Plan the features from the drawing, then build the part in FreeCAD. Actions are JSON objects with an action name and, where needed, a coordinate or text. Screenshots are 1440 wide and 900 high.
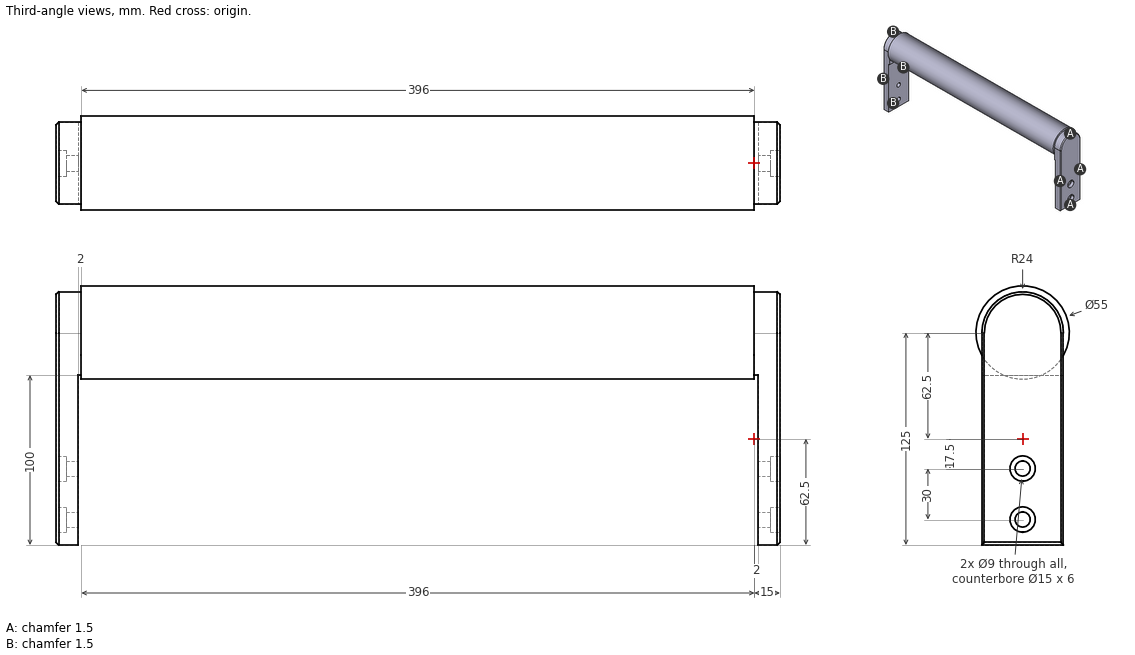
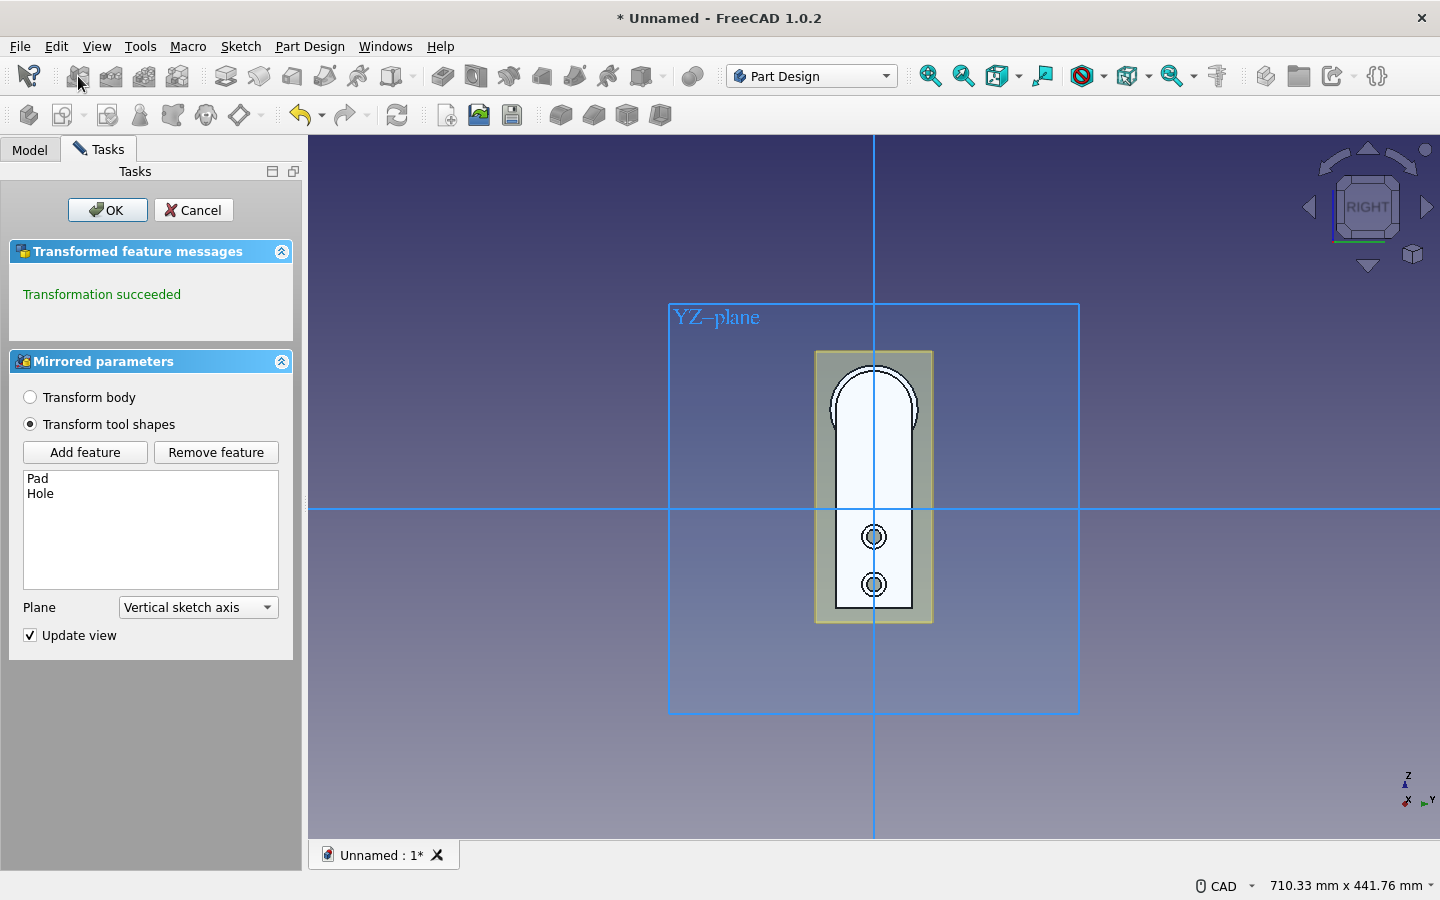
{"action": "left_click", "coordinate": [199, 608]}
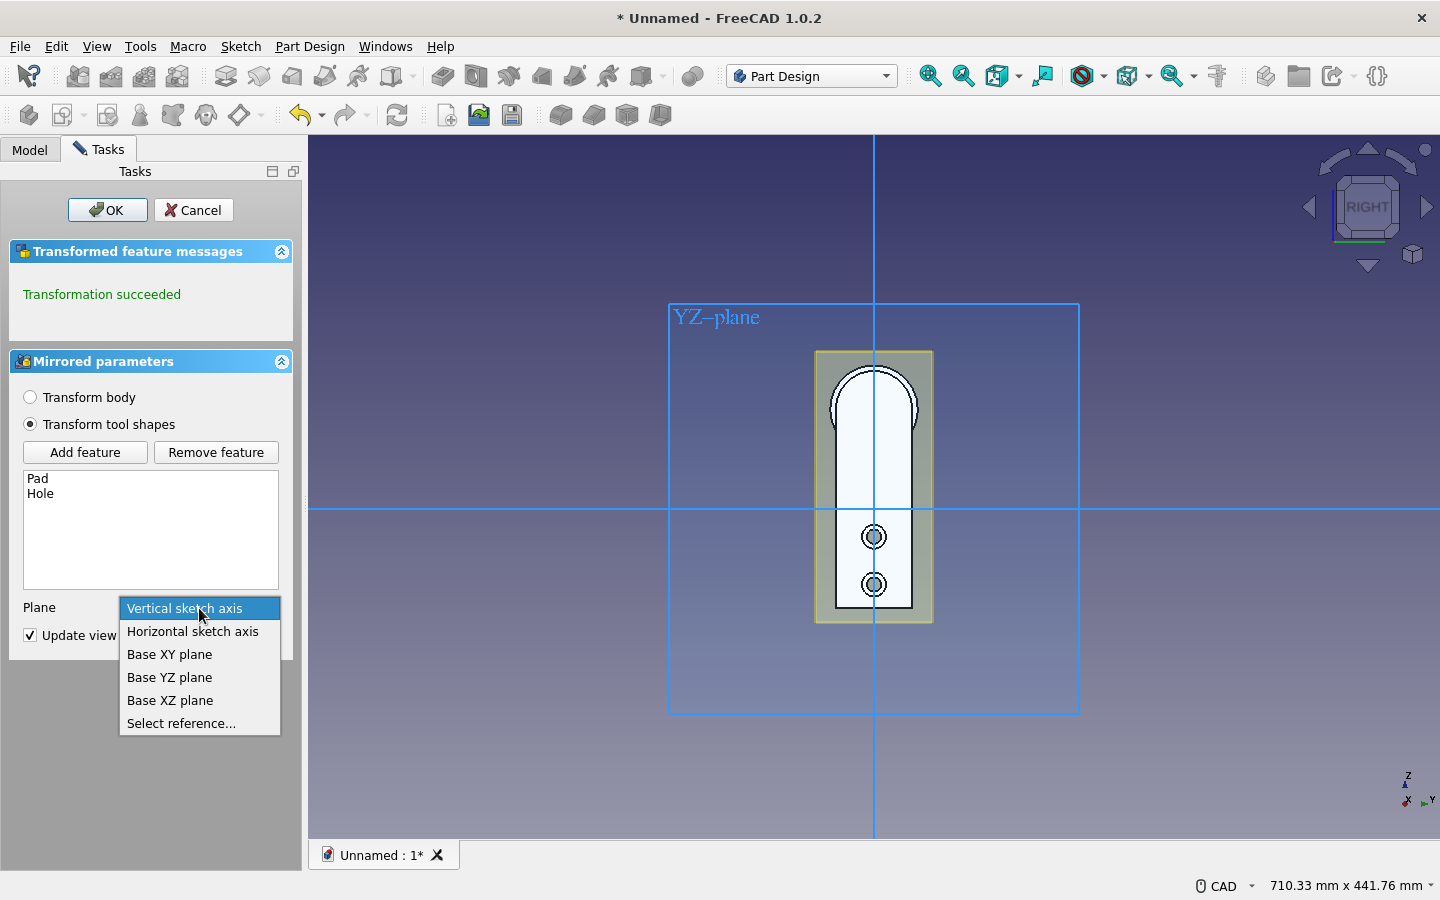
{"action": "left_click", "coordinate": [198, 724]}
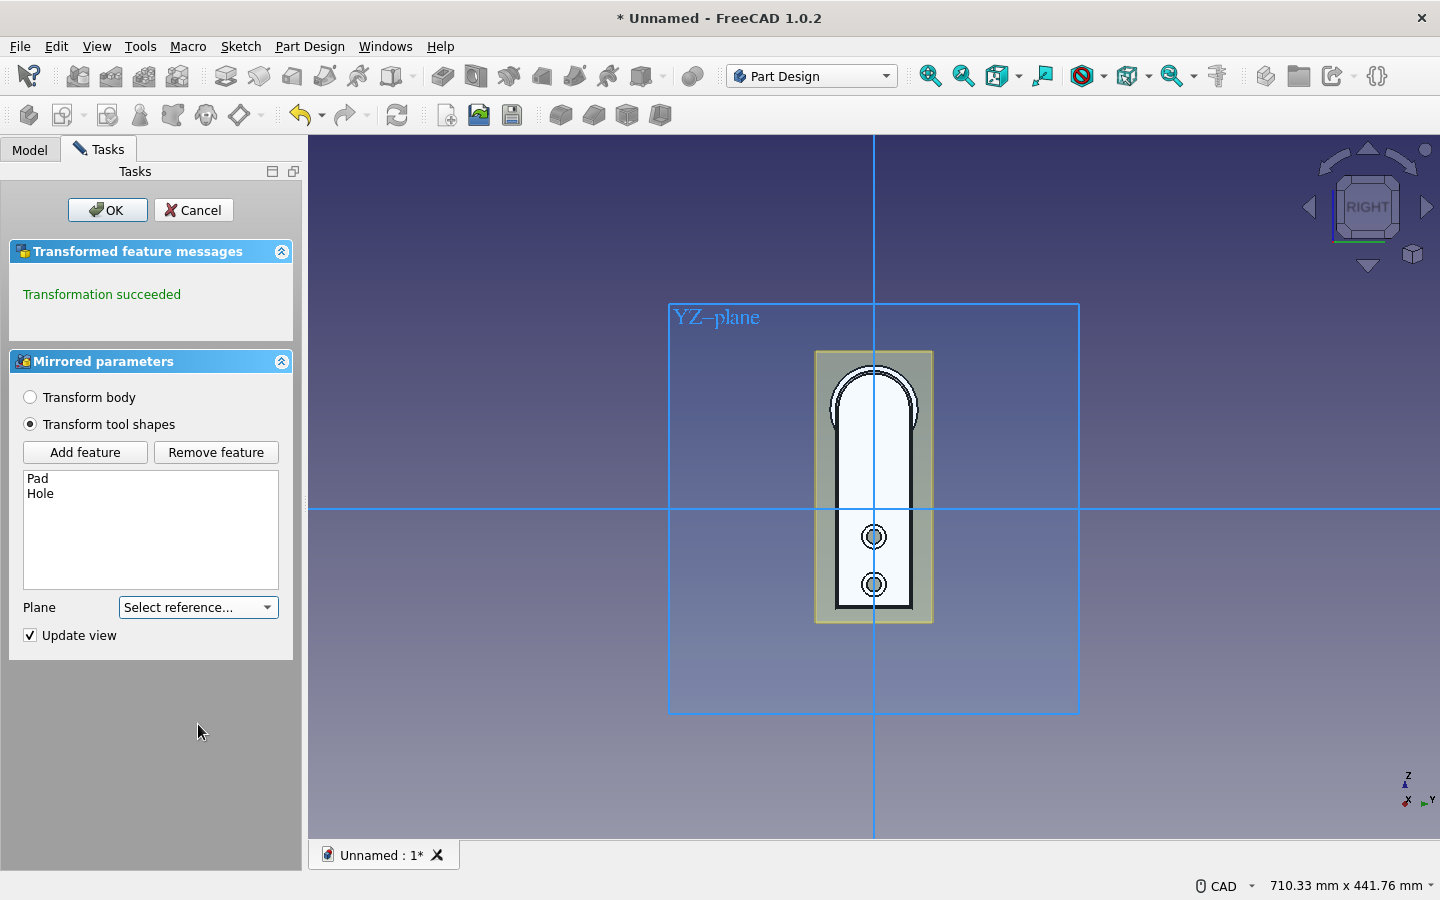
{"action": "left_click", "coordinate": [30, 149]}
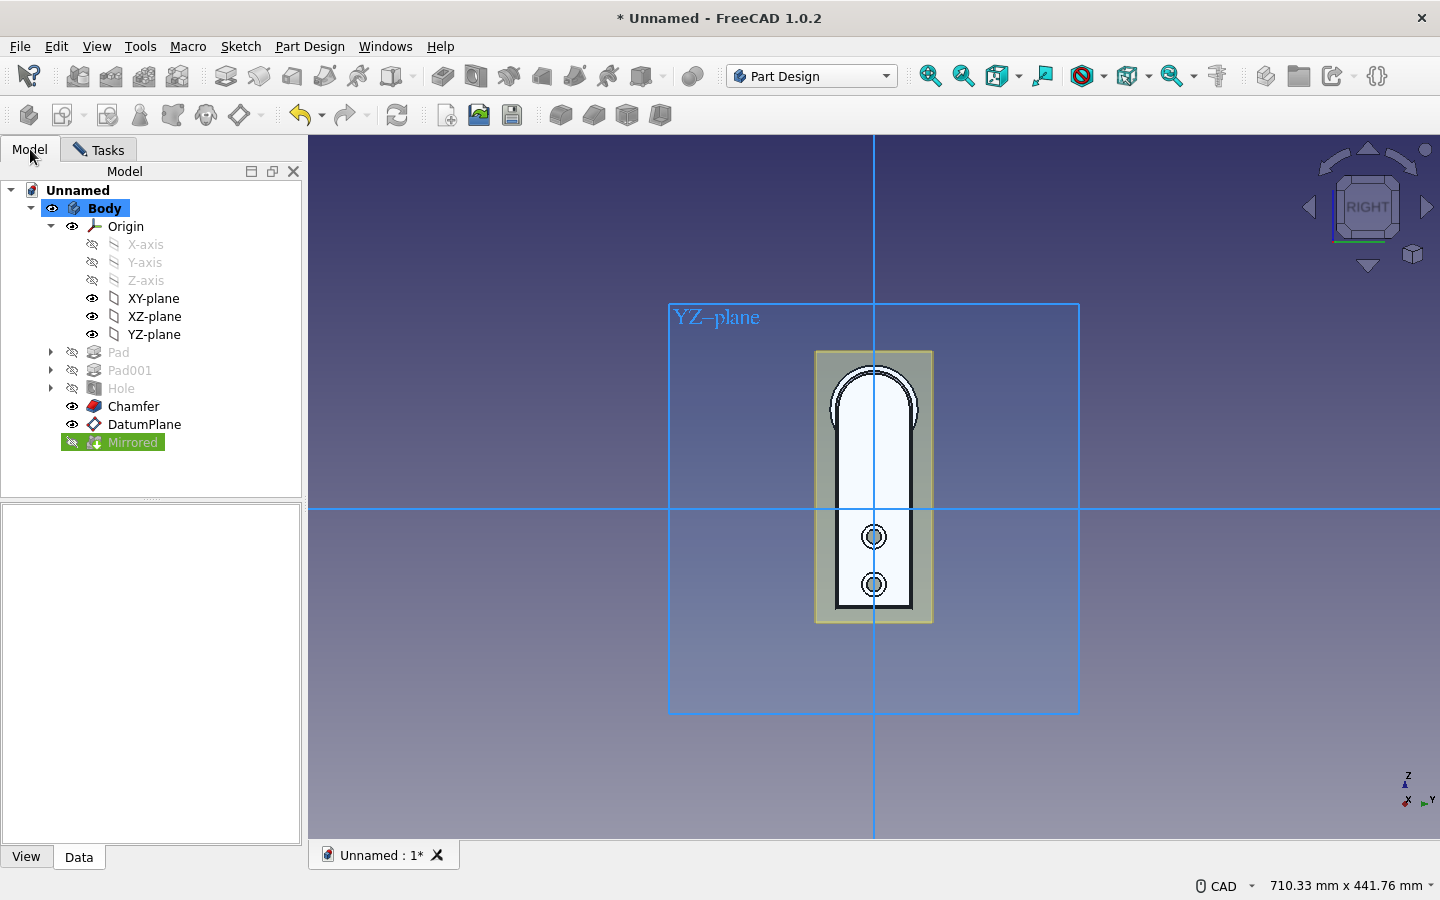
{"action": "left_click", "coordinate": [117, 424]}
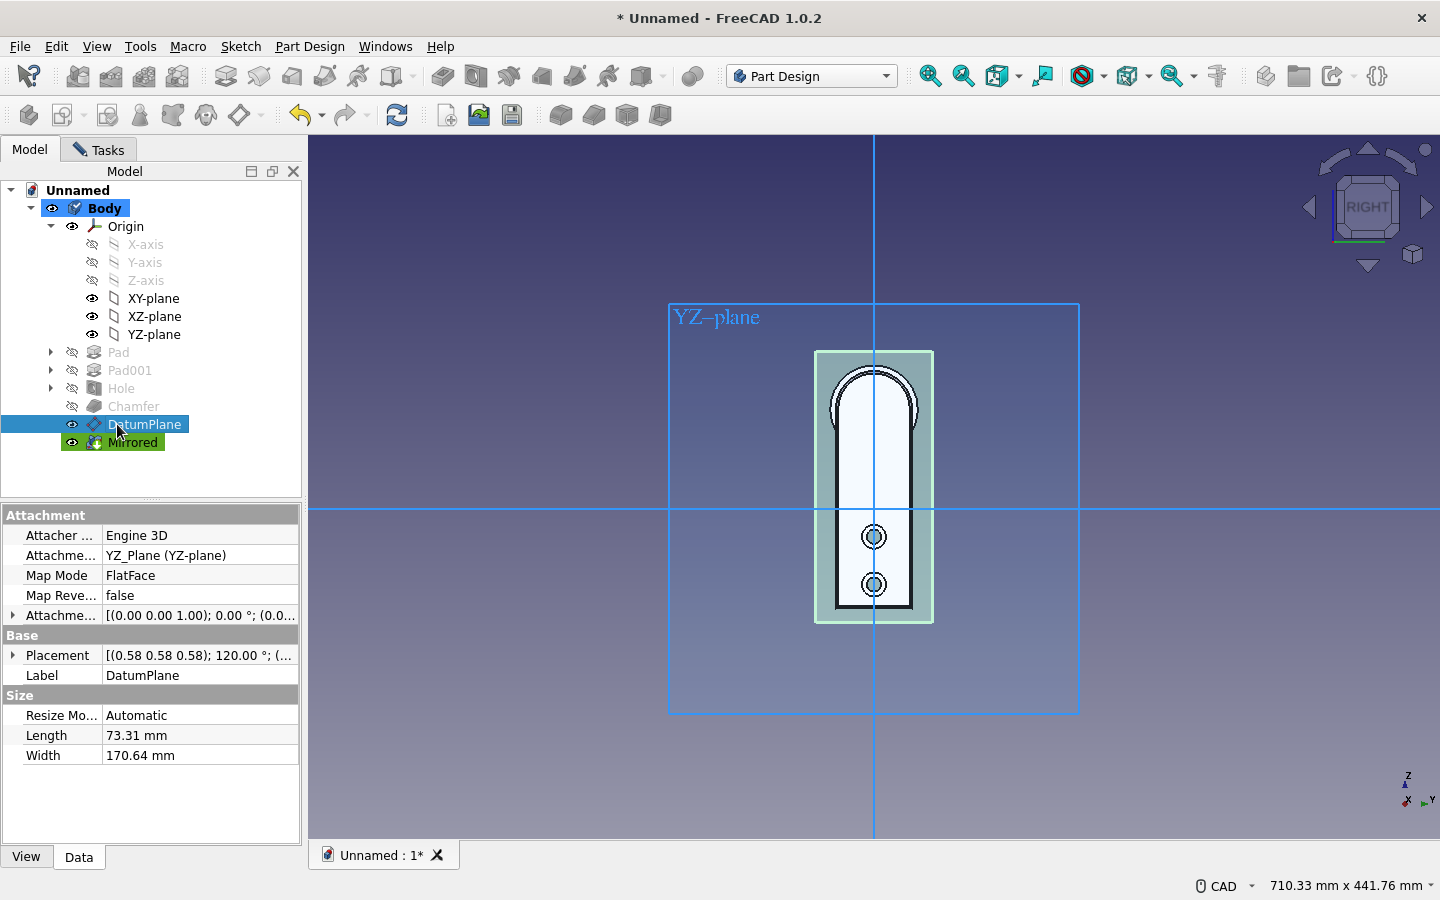
{"action": "left_click", "coordinate": [98, 149]}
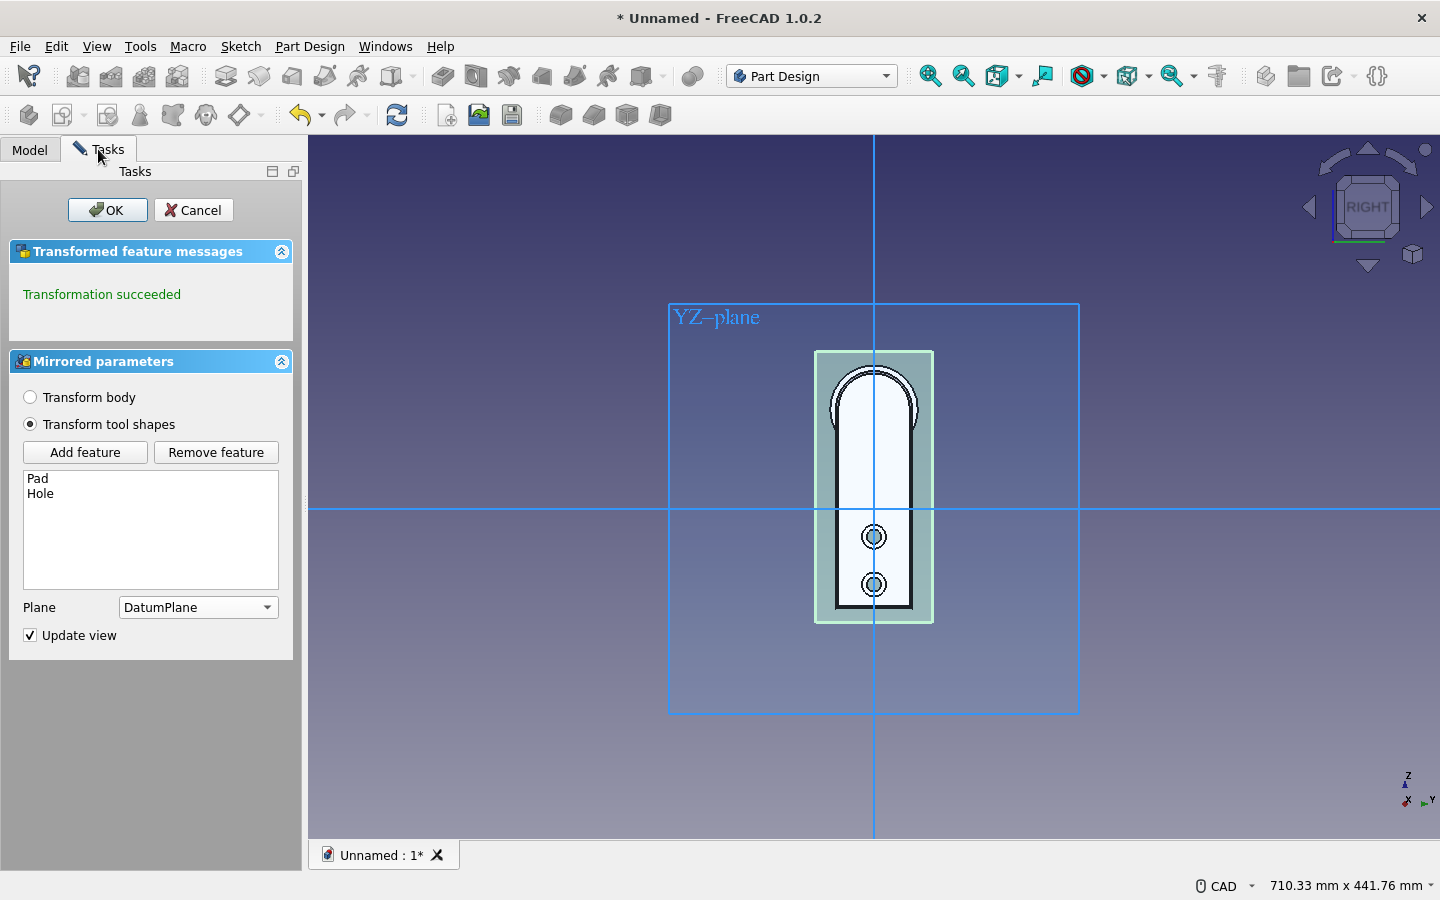
{"action": "left_click", "coordinate": [108, 210]}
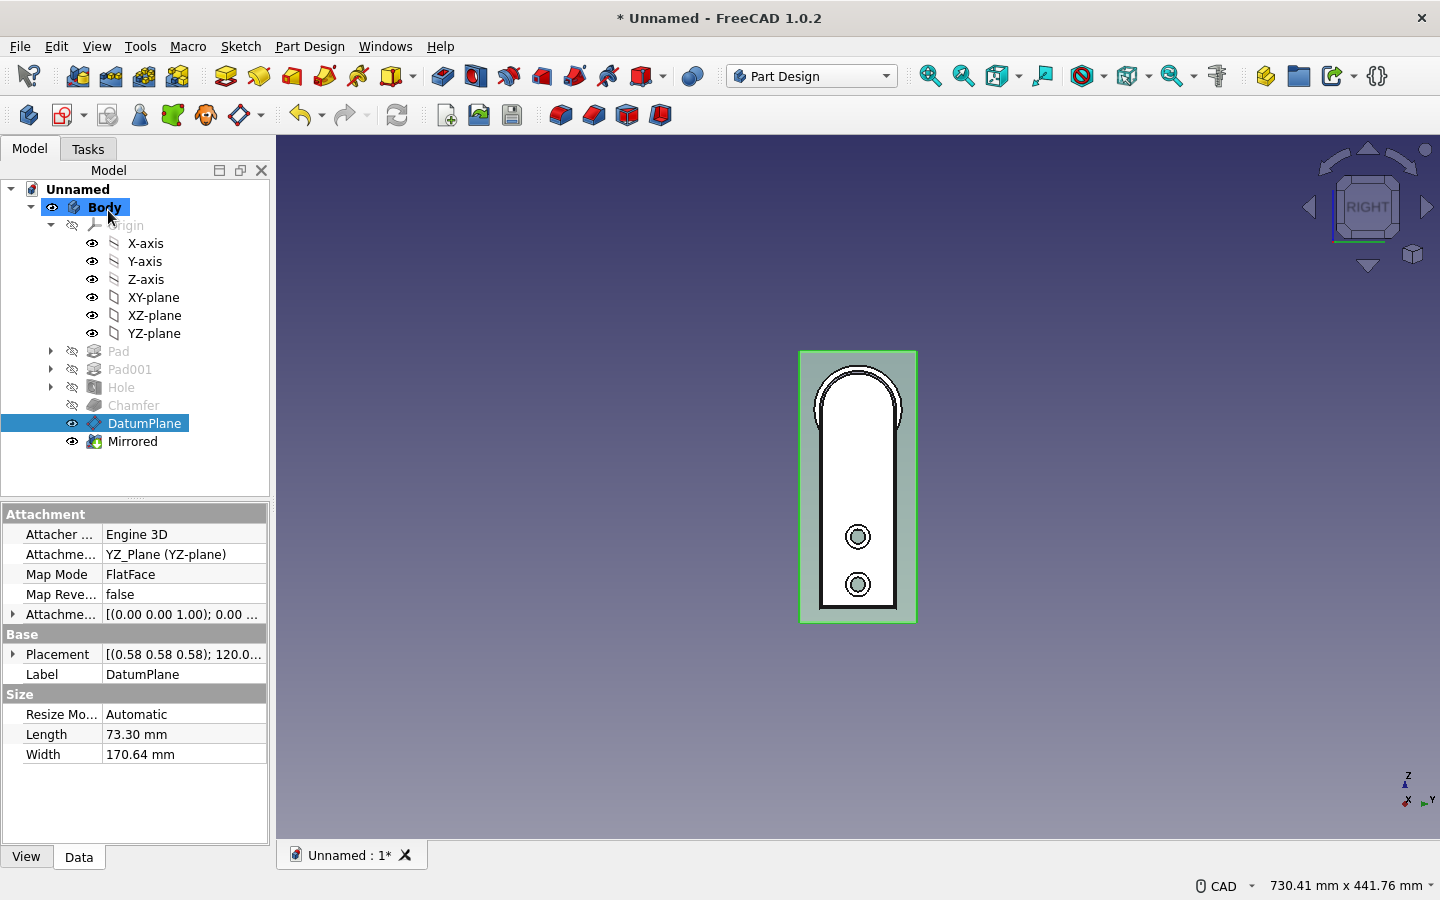
{"action": "left_click", "coordinate": [117, 423]}
{"action": "key", "text": "space"}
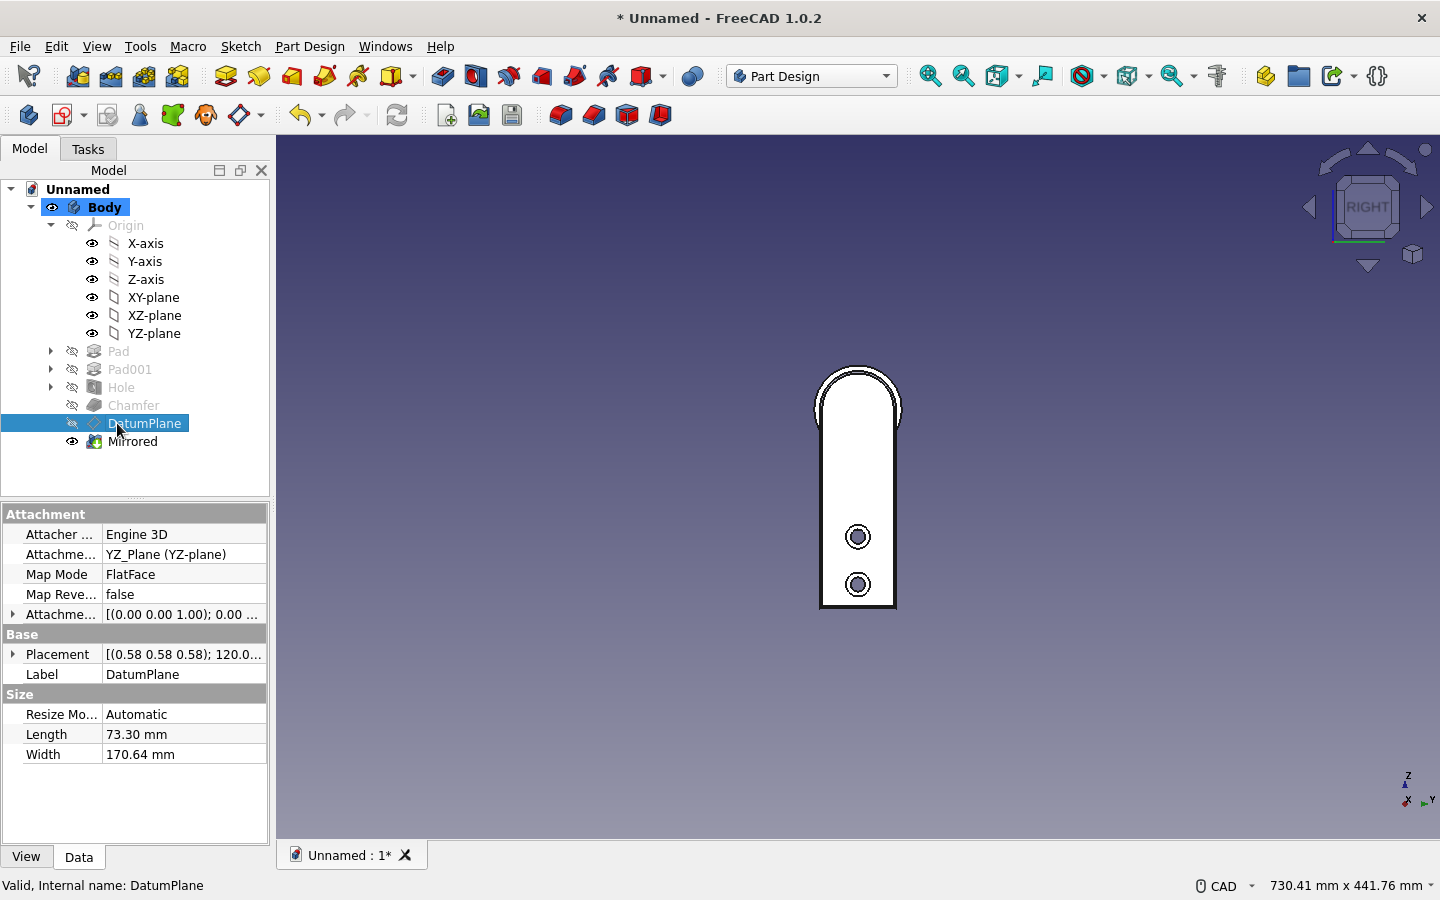
{"action": "left_click", "coordinate": [931, 76]}